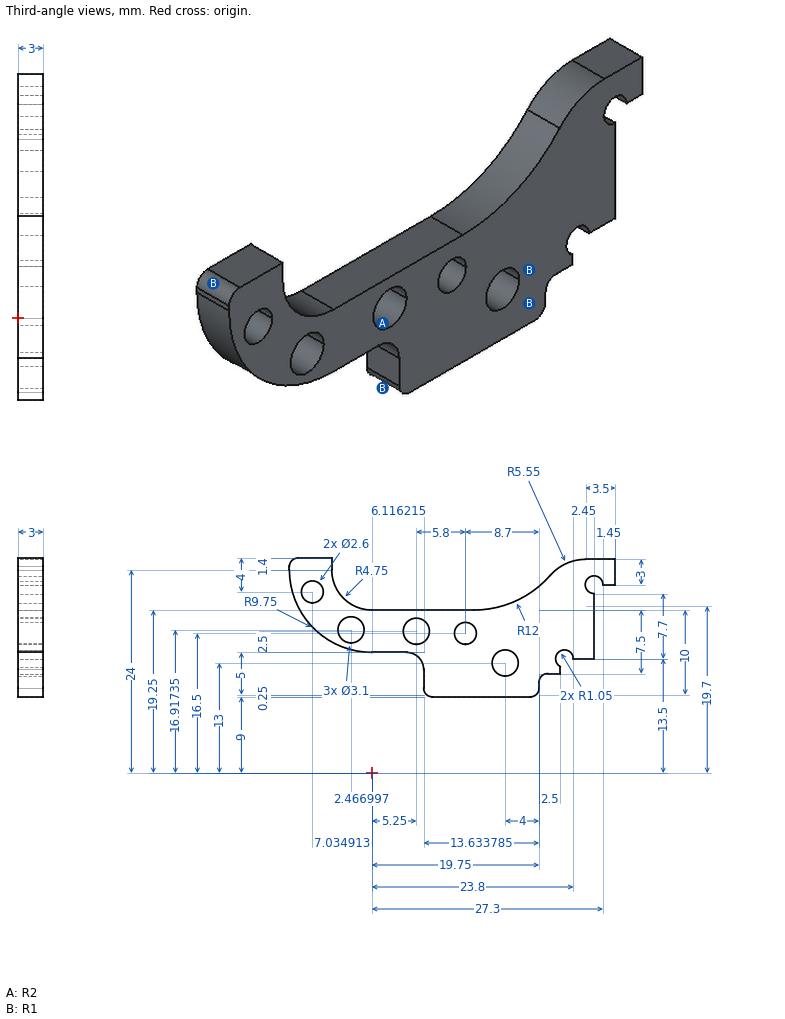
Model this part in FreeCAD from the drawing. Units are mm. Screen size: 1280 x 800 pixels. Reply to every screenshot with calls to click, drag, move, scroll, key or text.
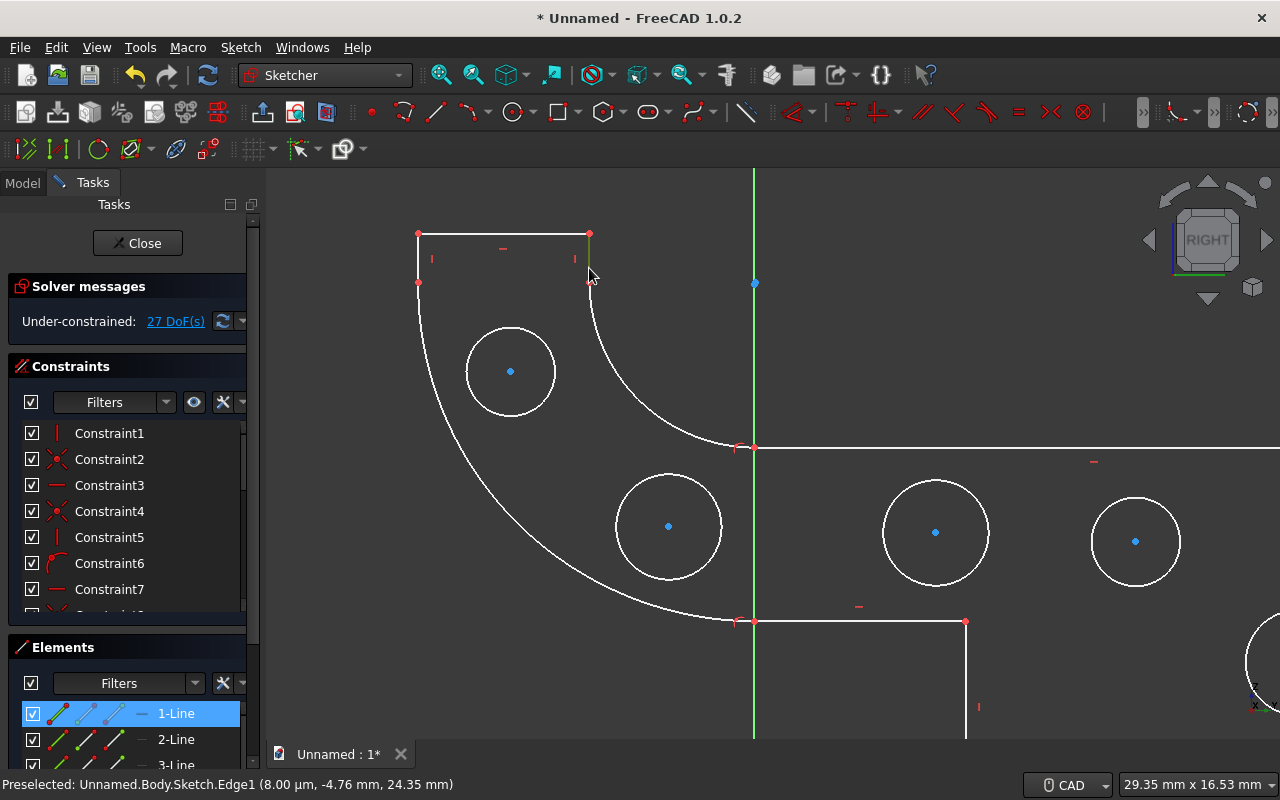
click(608, 357)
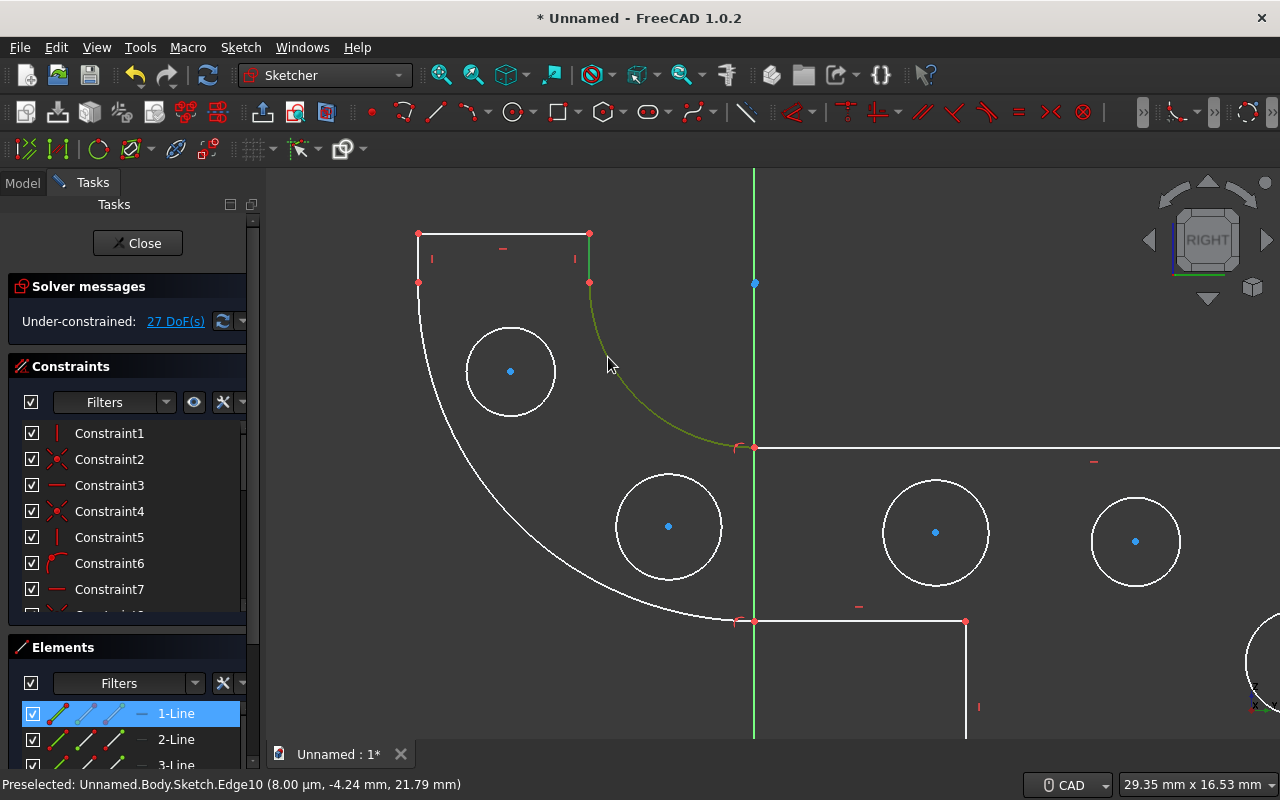
key(t)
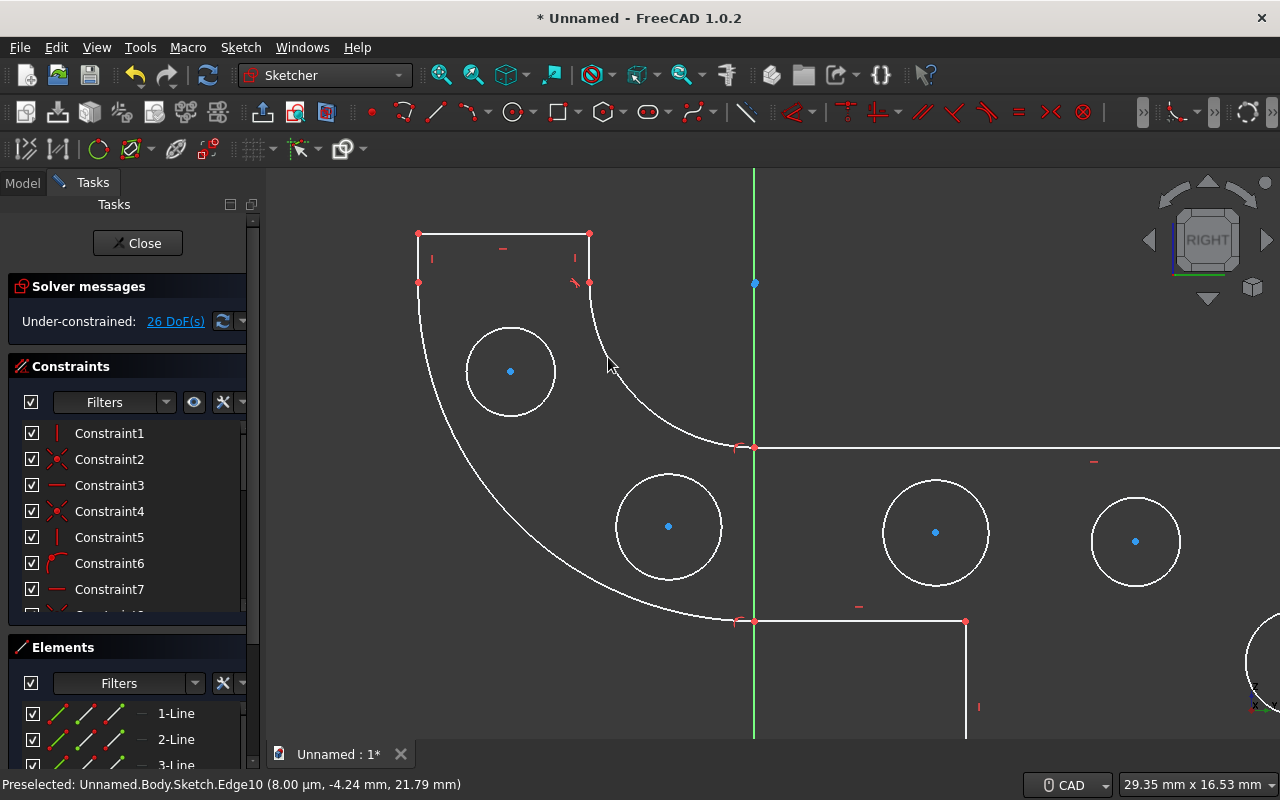
click(418, 249)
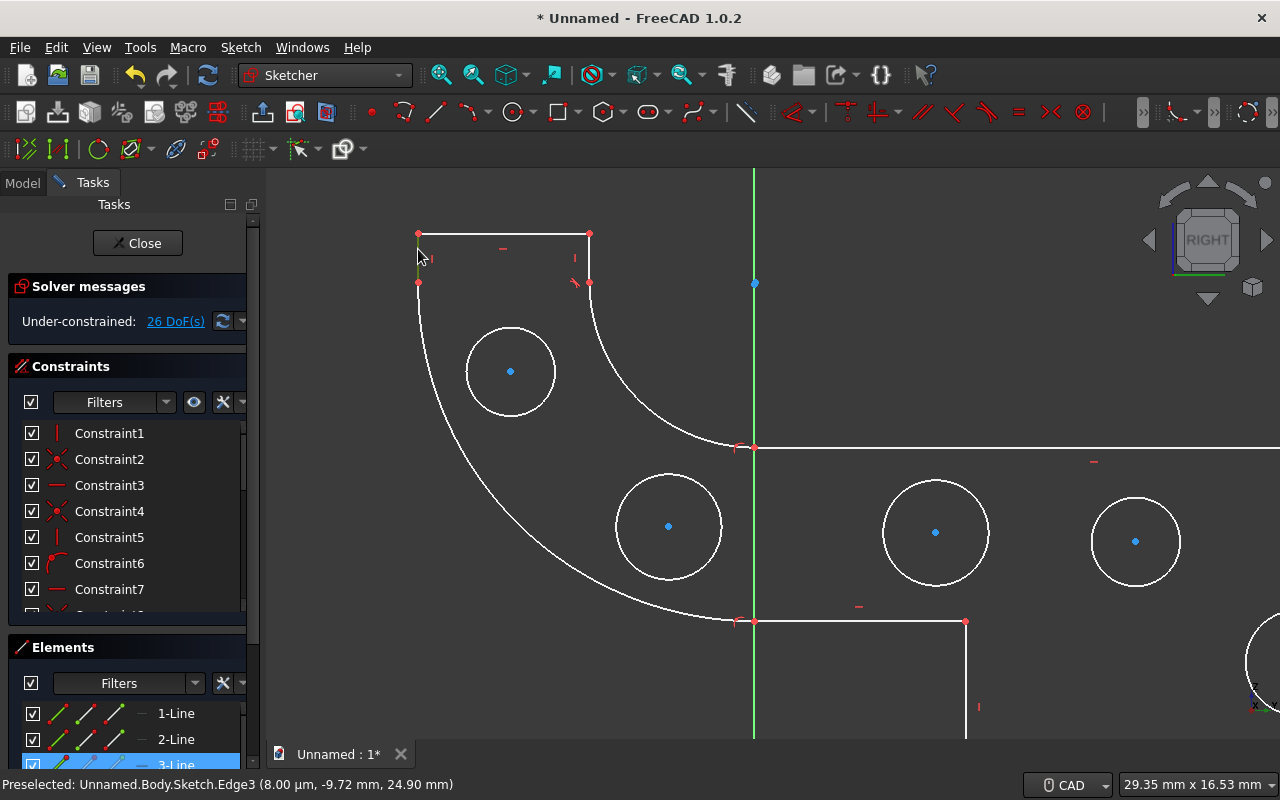
click(454, 436)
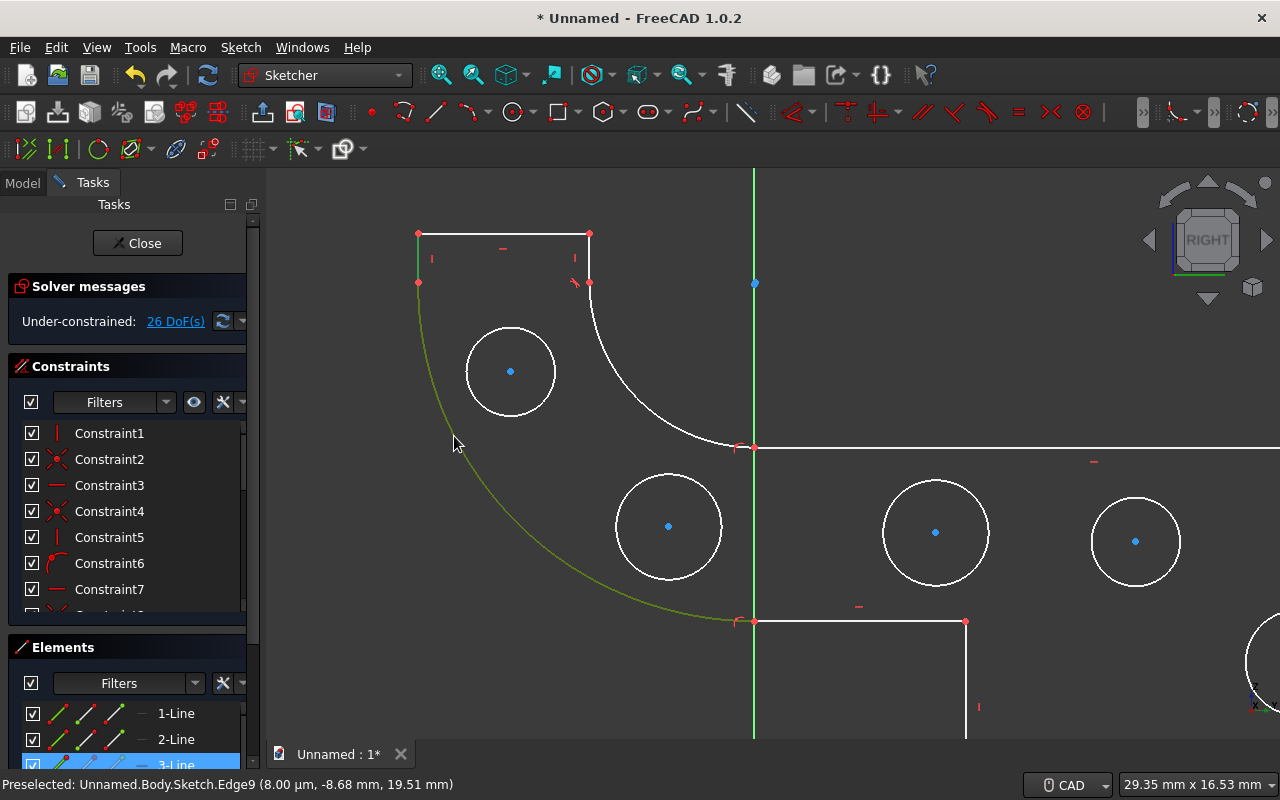
click(988, 112)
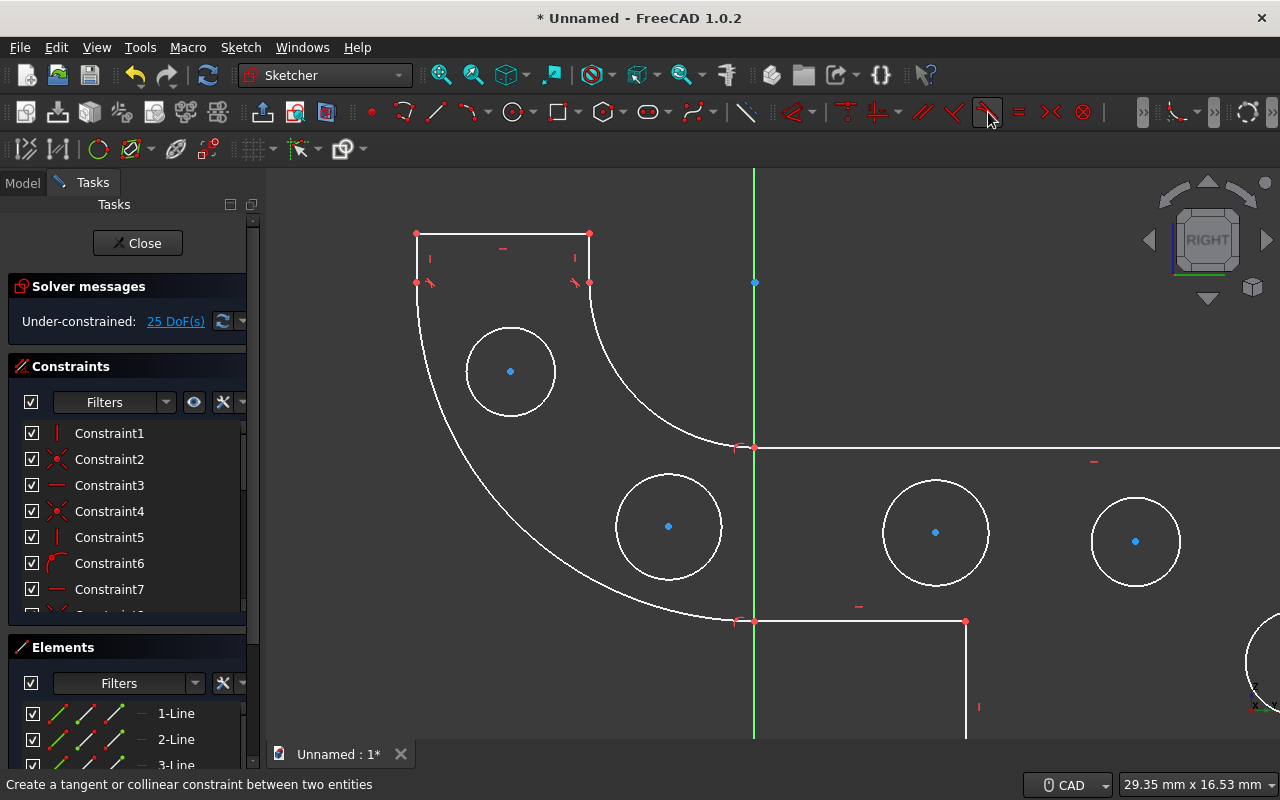
click(818, 621)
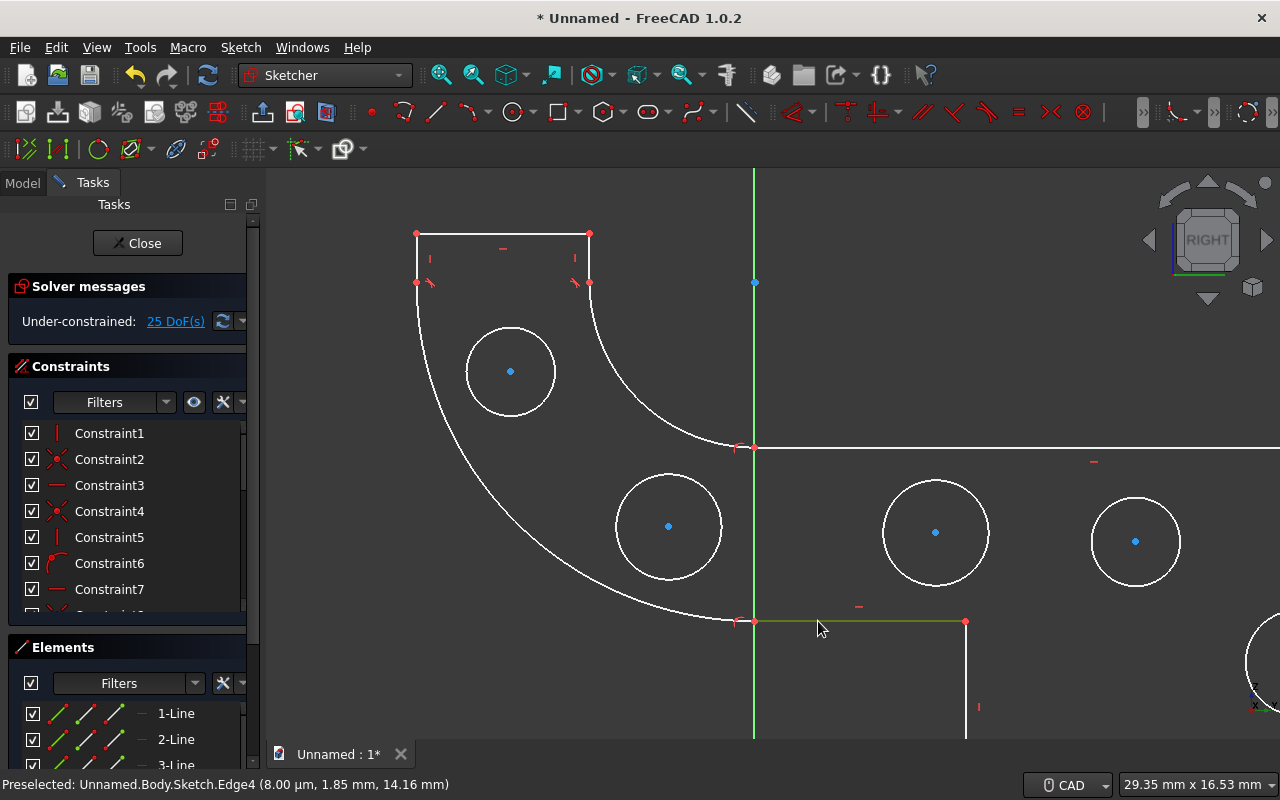
click(453, 436)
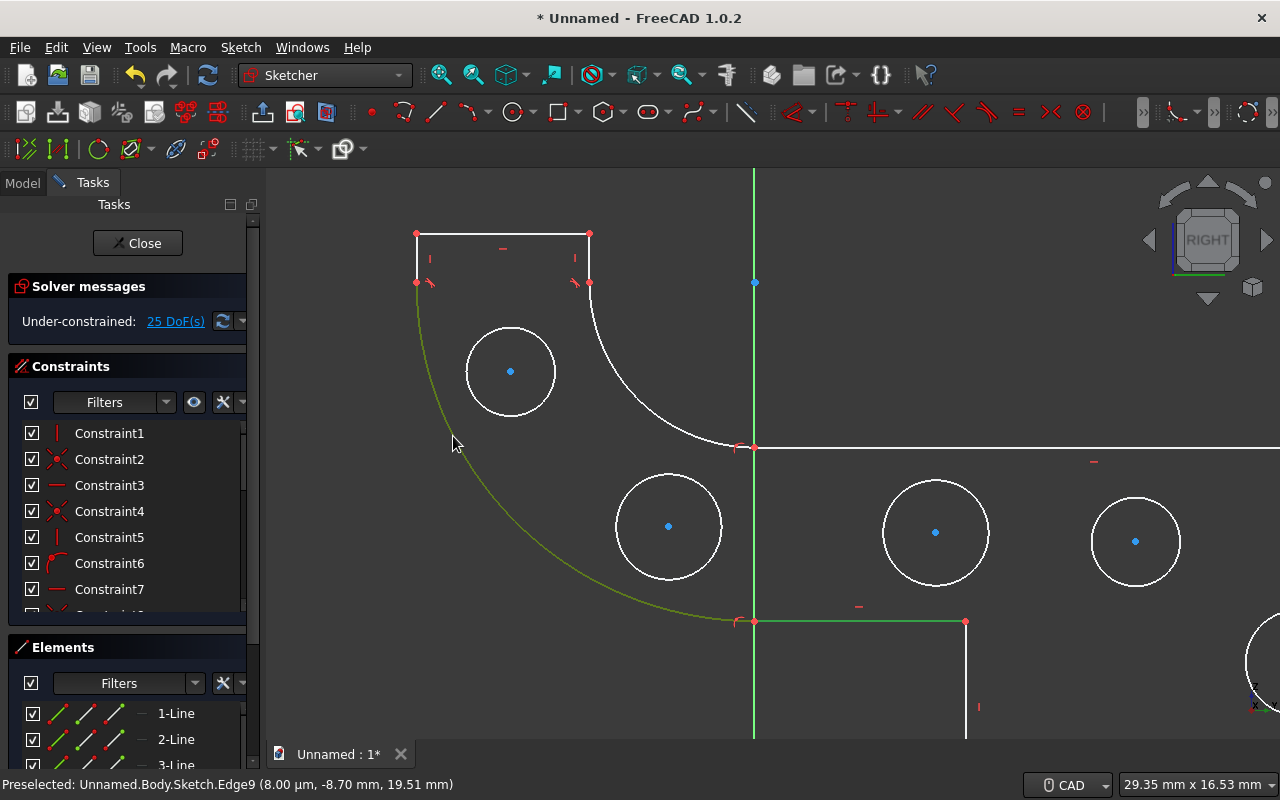
key(t)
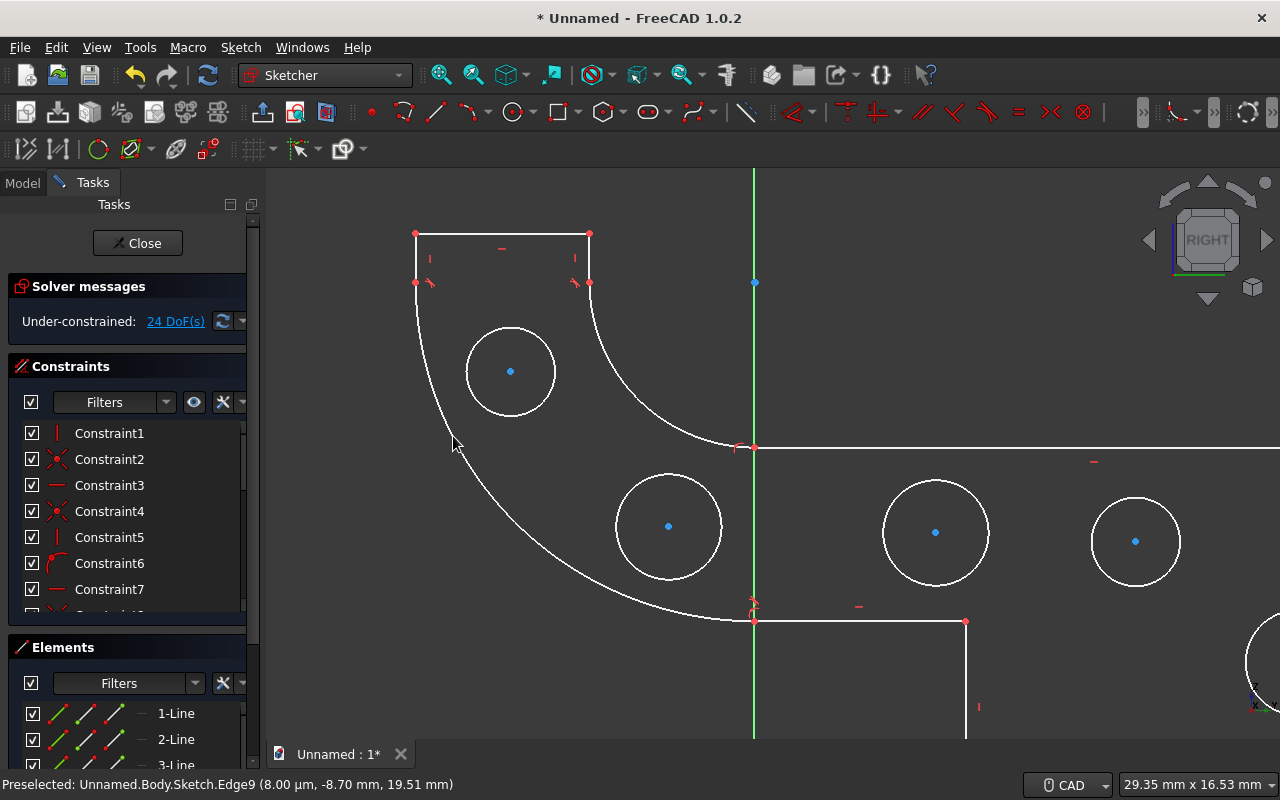
click(958, 448)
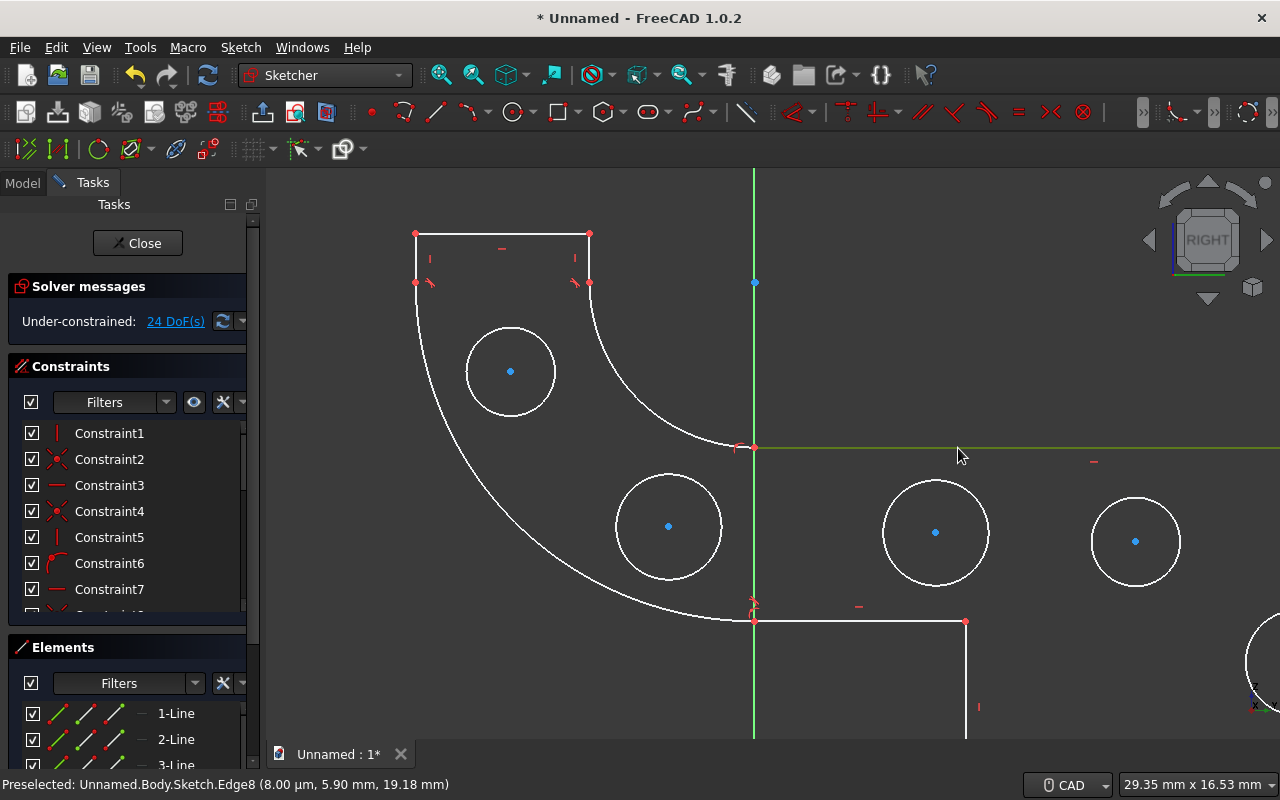
click(607, 357)